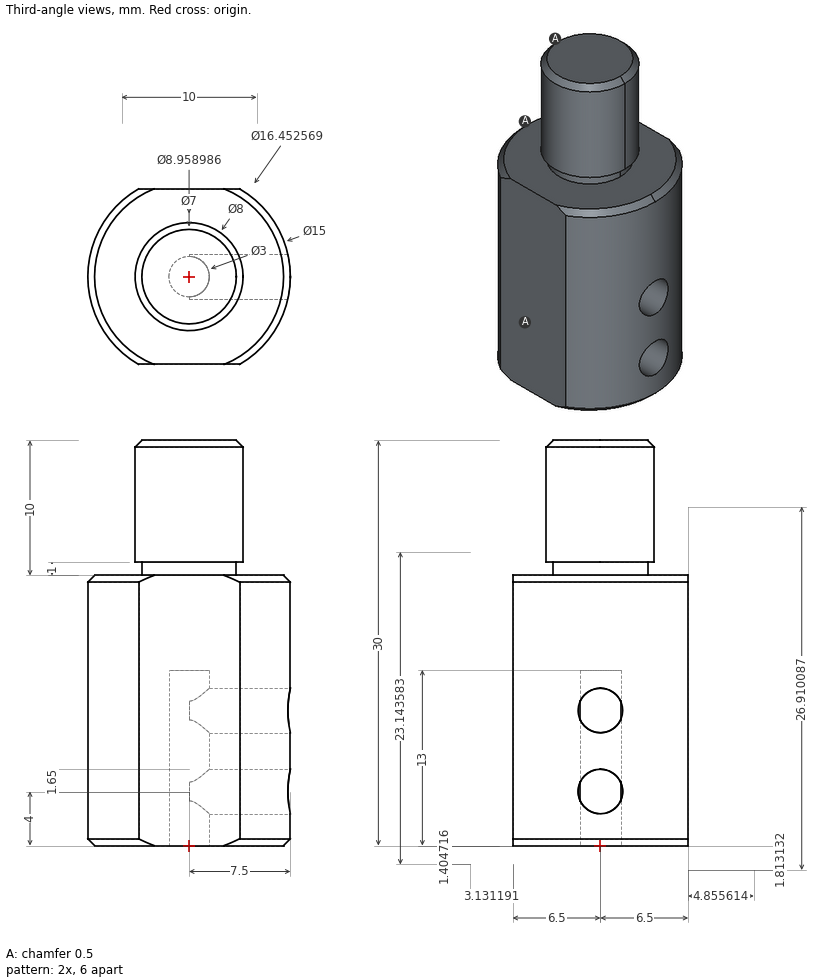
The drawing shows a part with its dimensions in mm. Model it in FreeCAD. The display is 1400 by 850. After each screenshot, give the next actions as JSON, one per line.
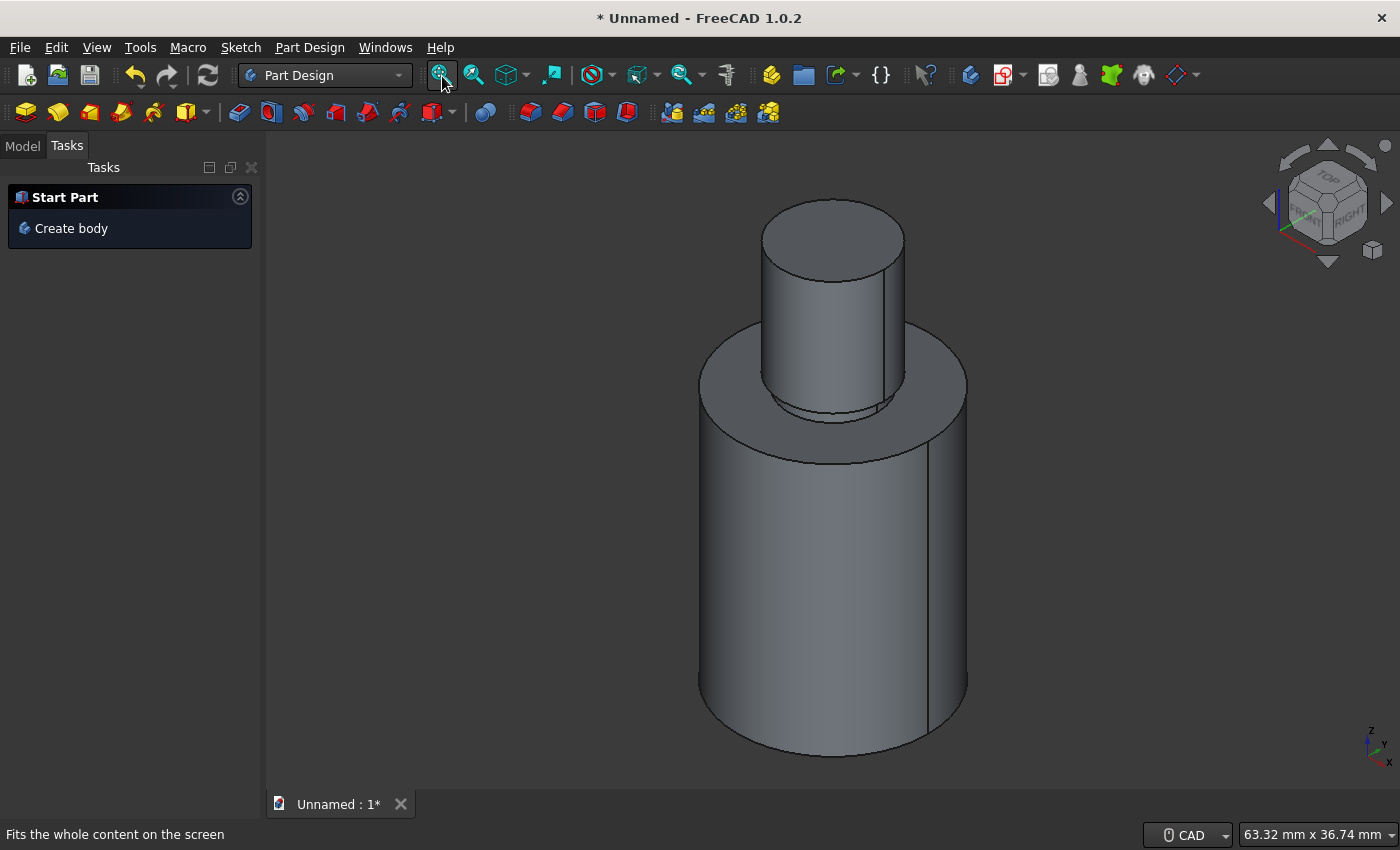
{"action": "left_click", "coordinate": [713, 714]}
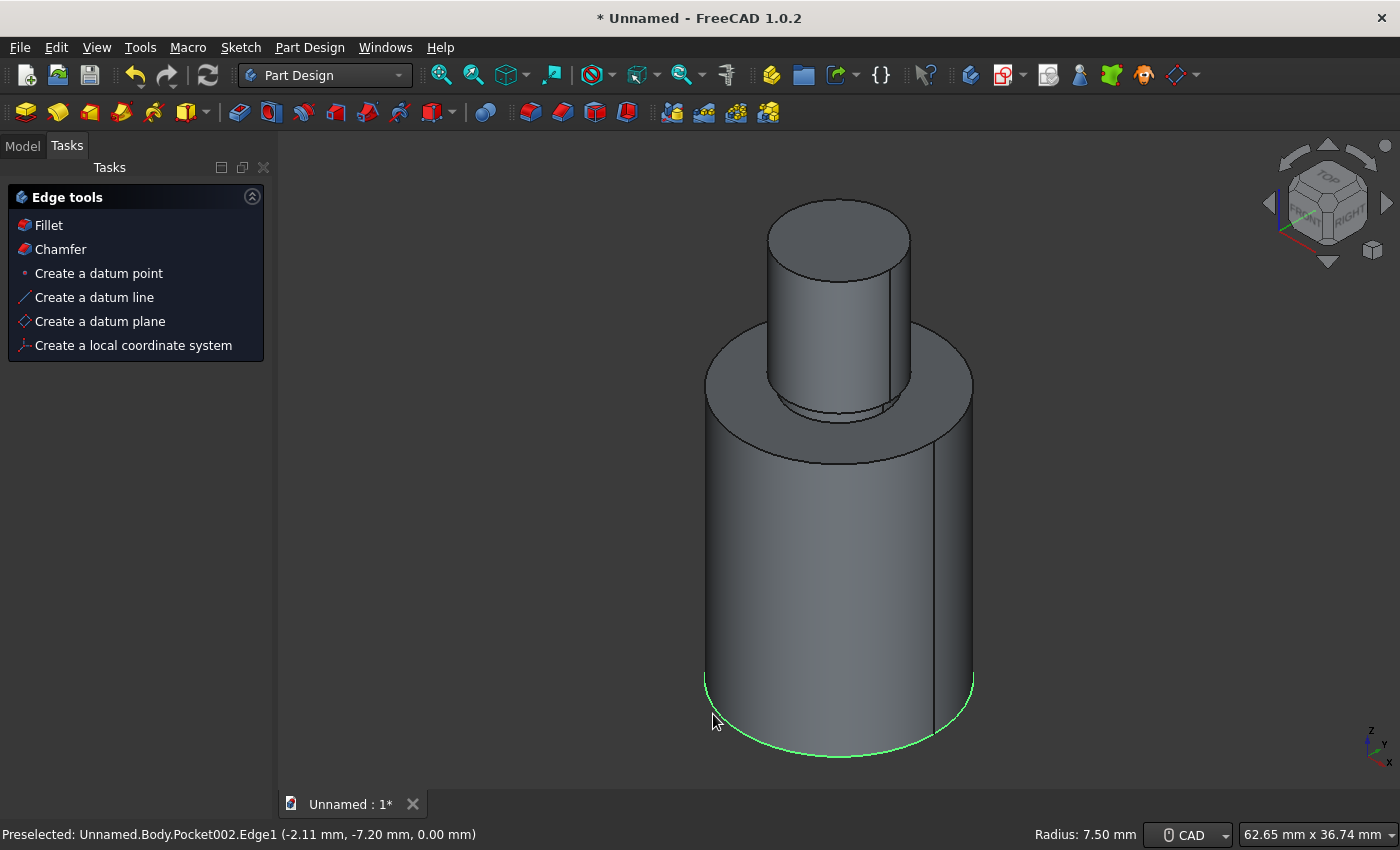
{"action": "left_click", "coordinate": [719, 421], "text": "ctrl"}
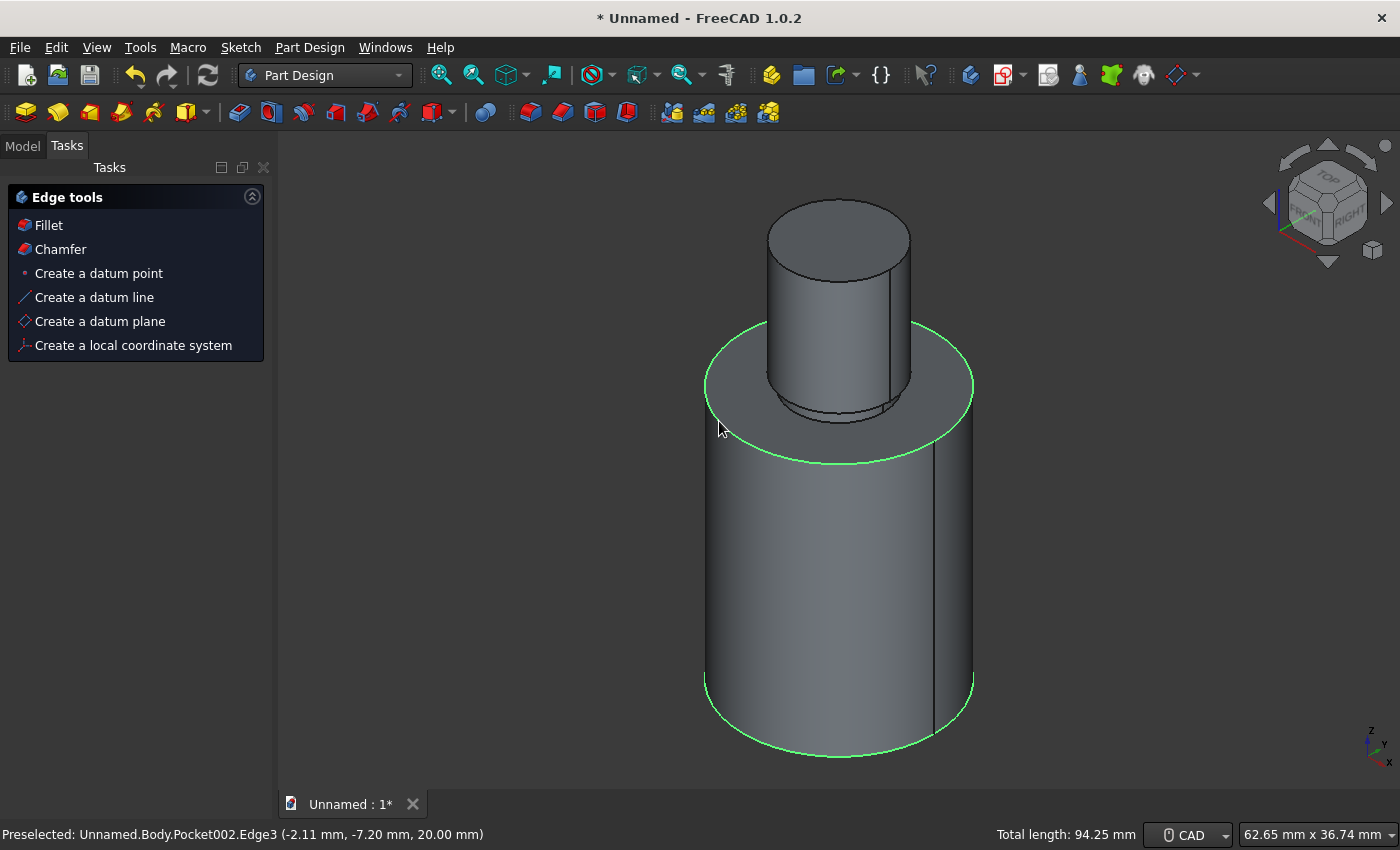
{"action": "left_click", "coordinate": [775, 258], "text": "ctrl"}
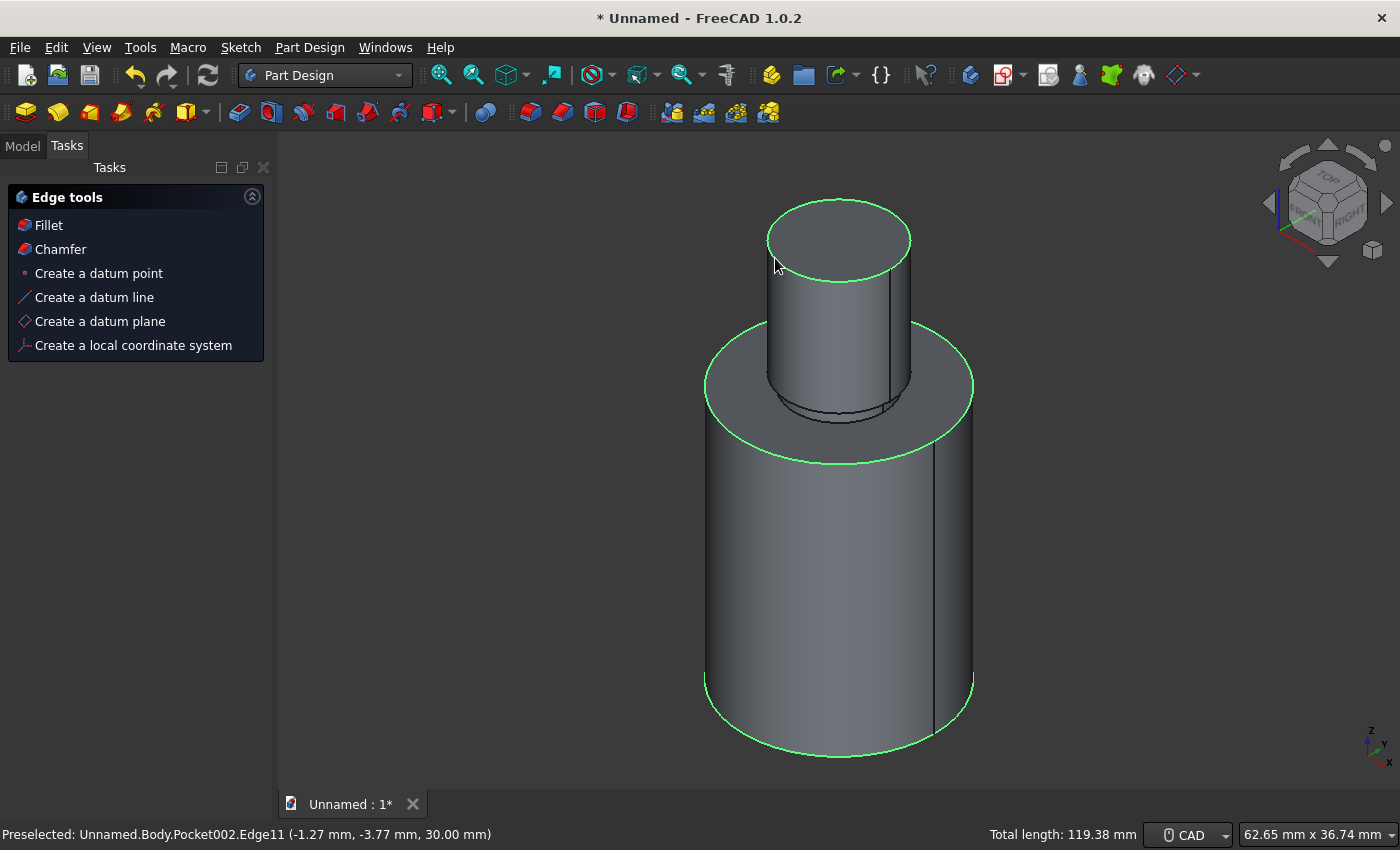
{"action": "left_click", "coordinate": [564, 112]}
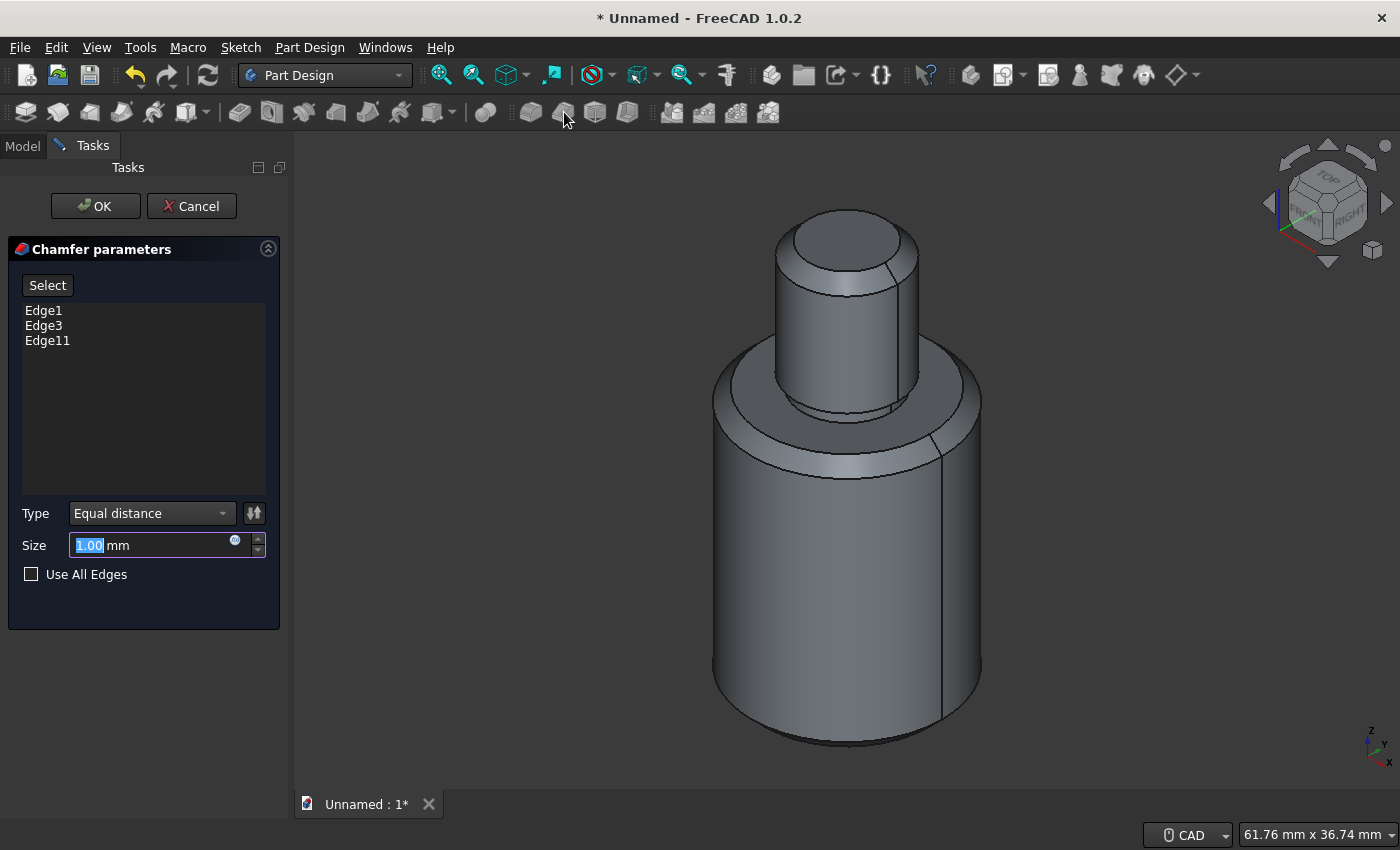
{"action": "type", "text": "0.5"}
{"action": "key", "text": "Tab"}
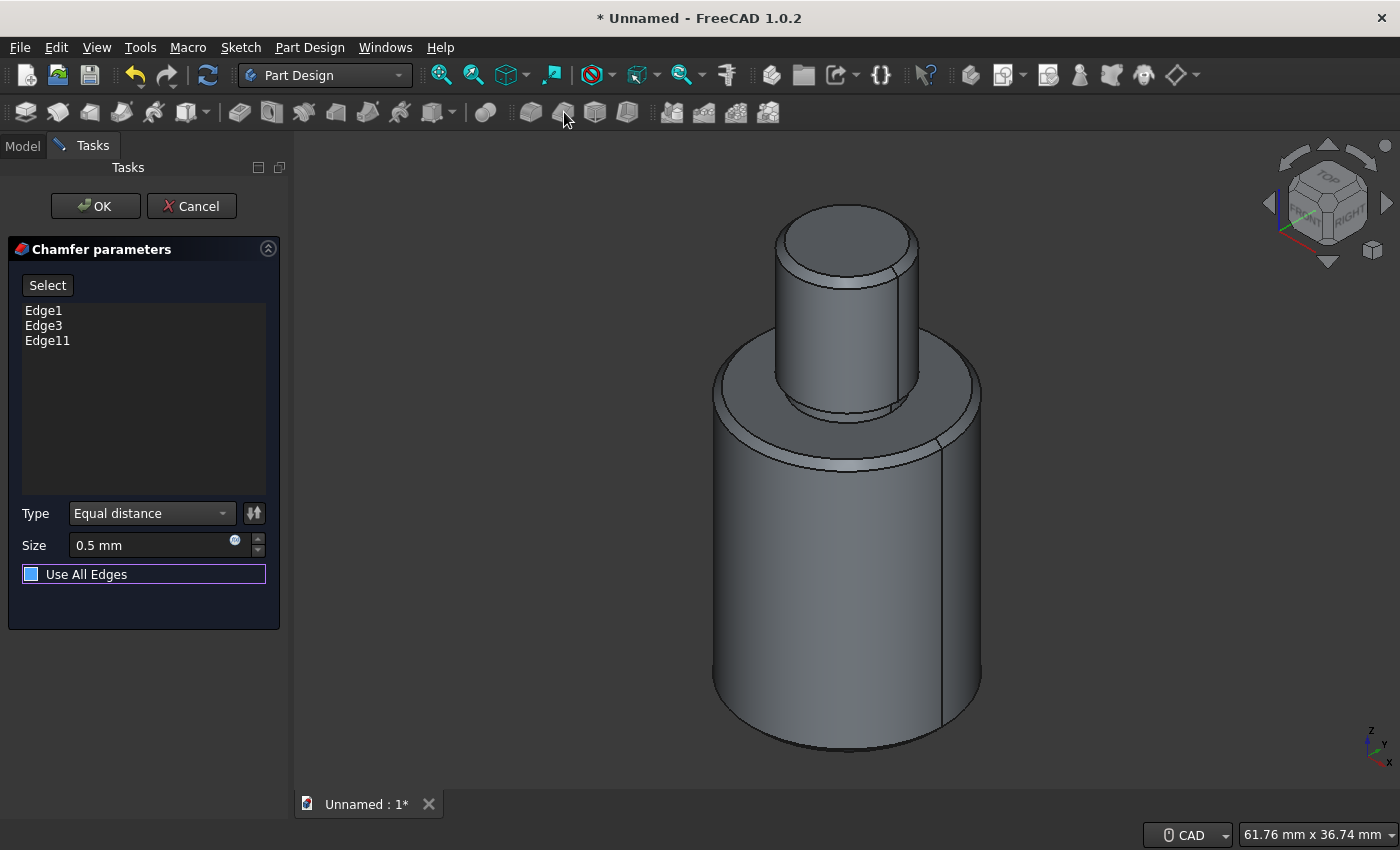
{"action": "left_click", "coordinate": [96, 206]}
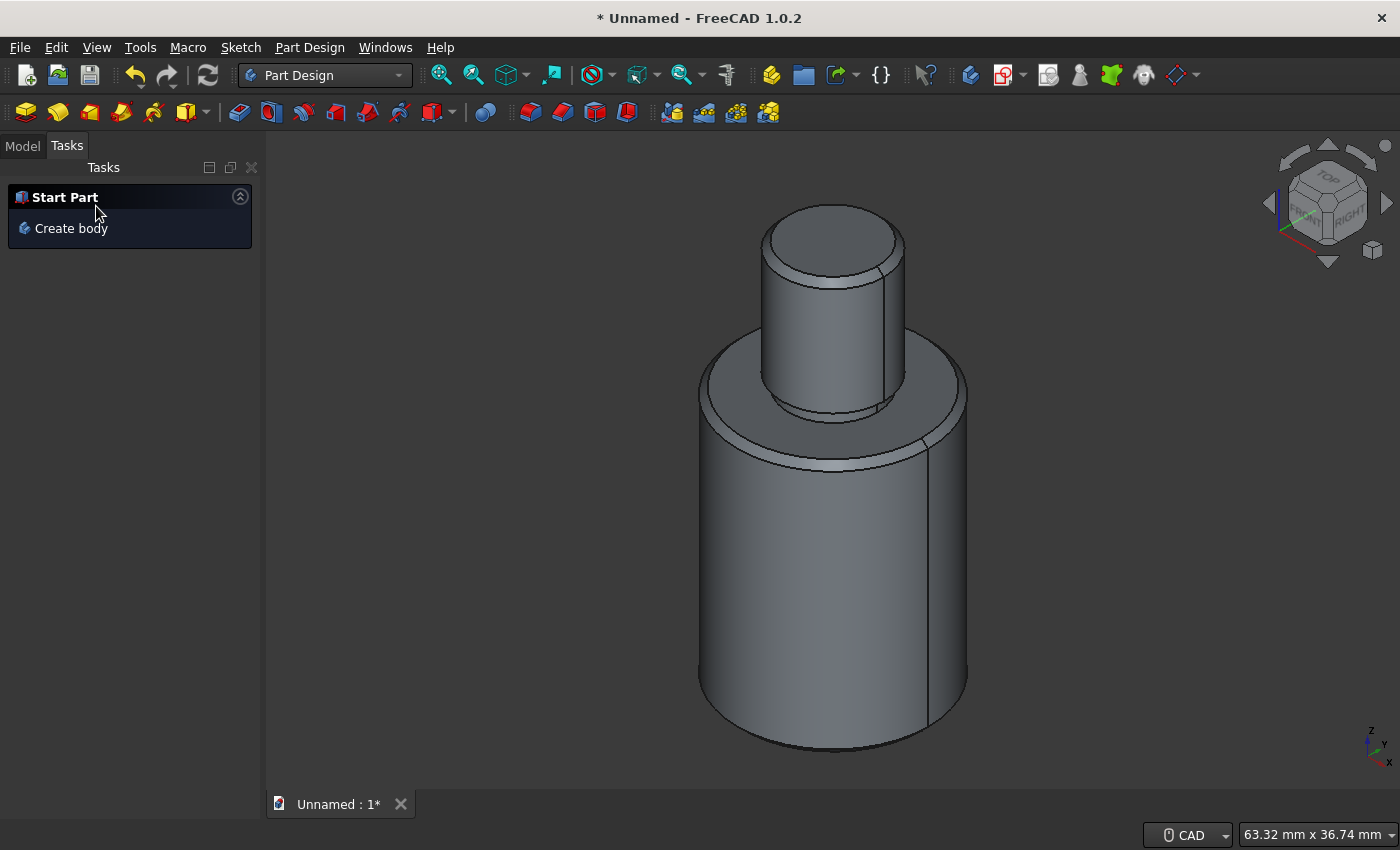
{"action": "left_click", "coordinate": [442, 76]}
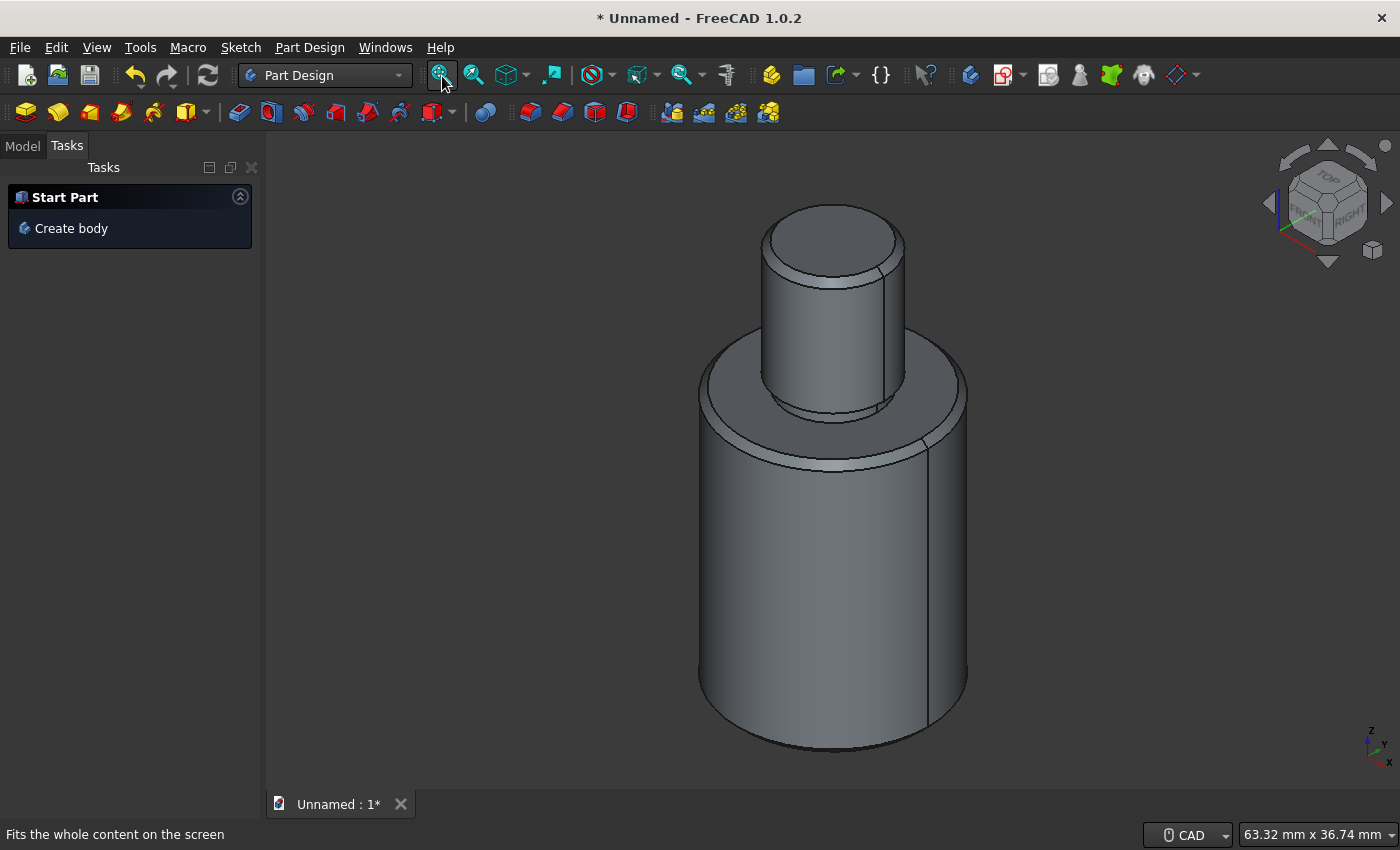
{"action": "left_click", "coordinate": [1004, 76]}